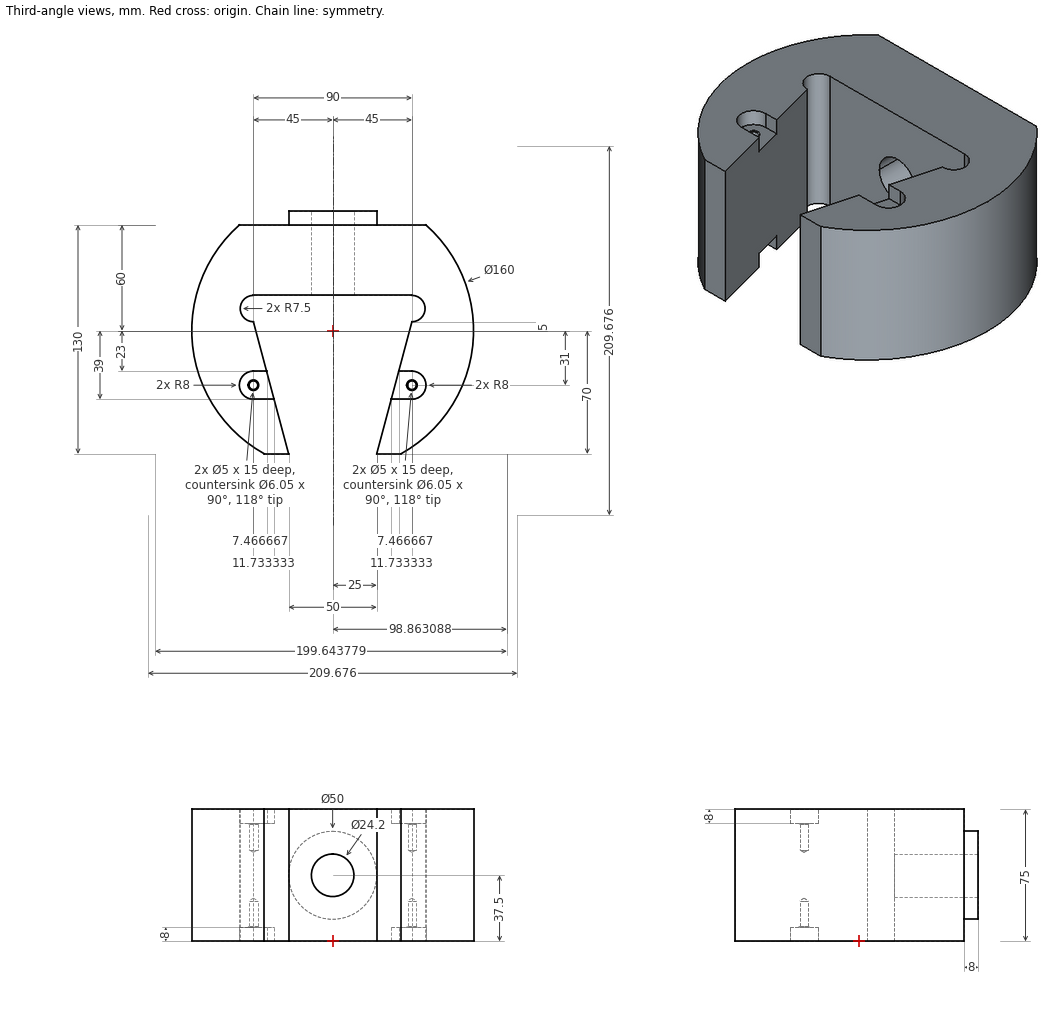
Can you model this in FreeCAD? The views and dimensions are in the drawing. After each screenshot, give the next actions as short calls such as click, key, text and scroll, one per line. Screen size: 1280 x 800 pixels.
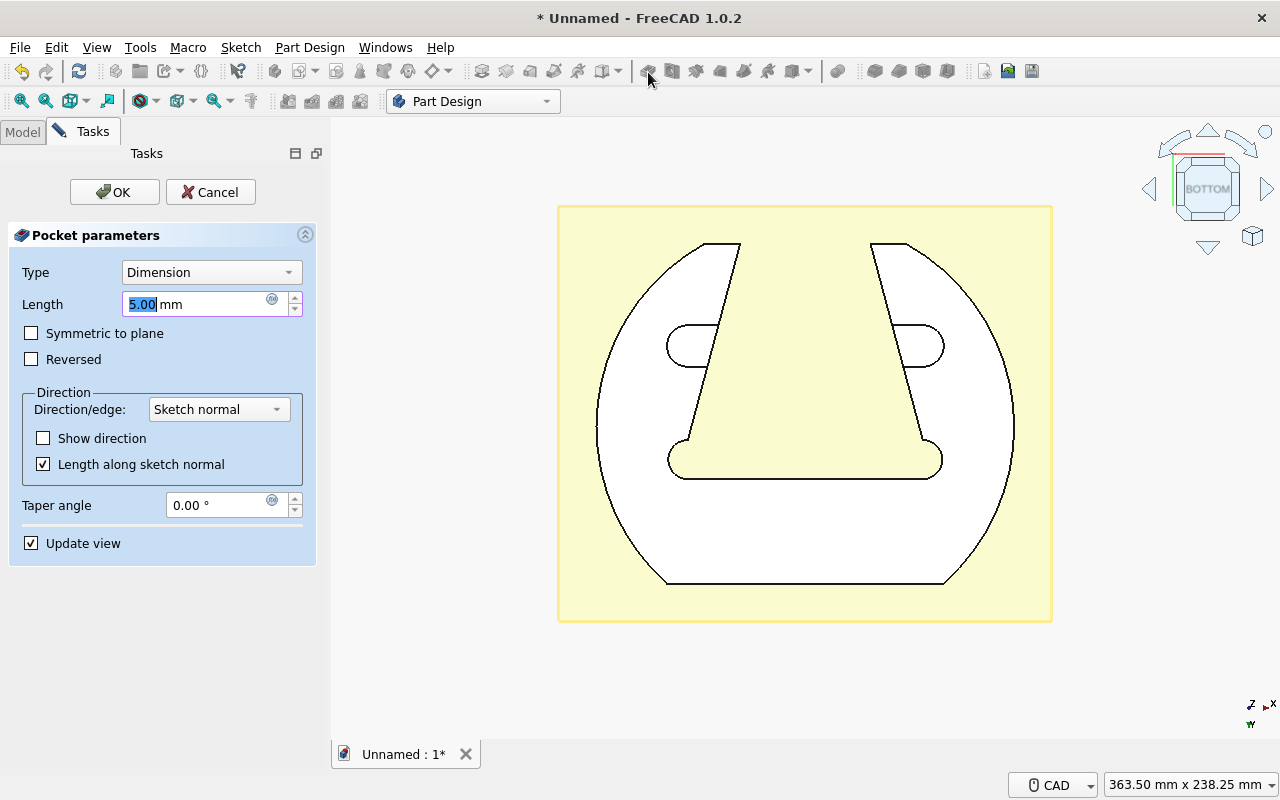
text(8)
key(Tab)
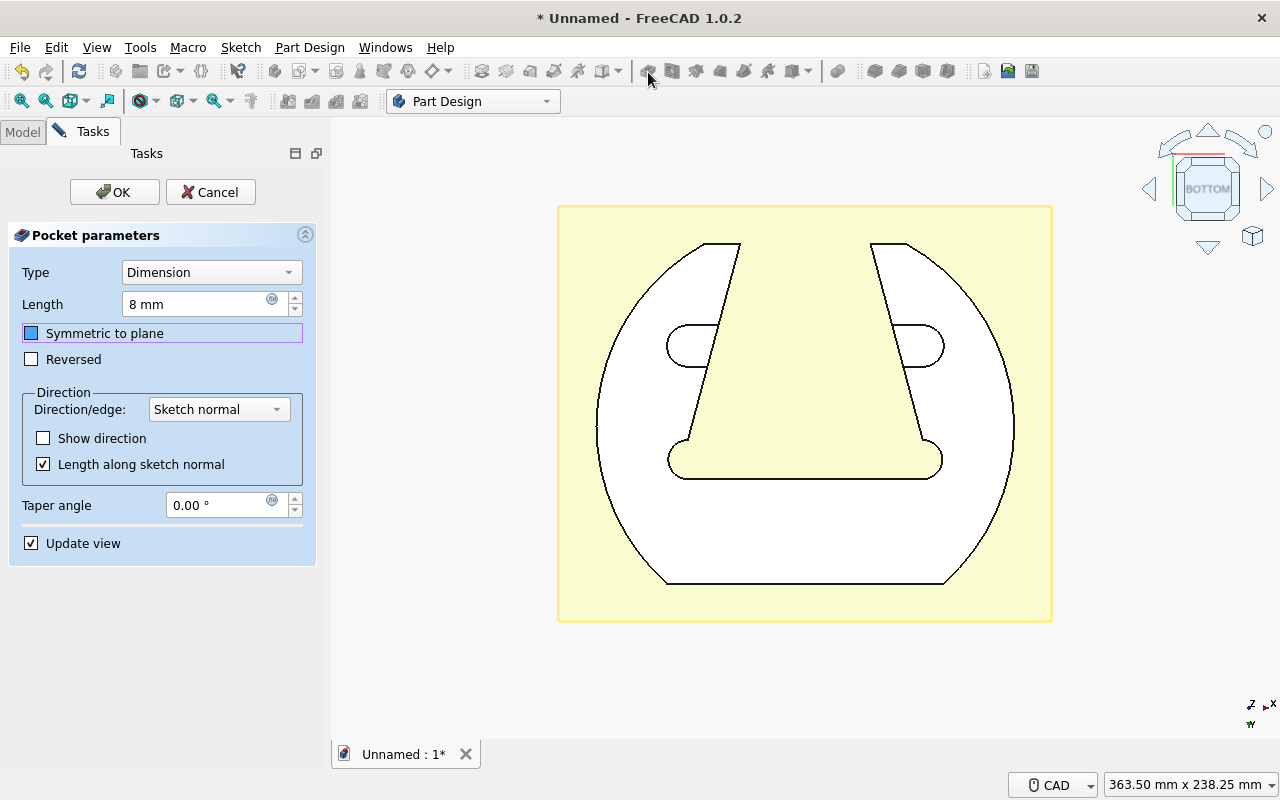
click(30, 359)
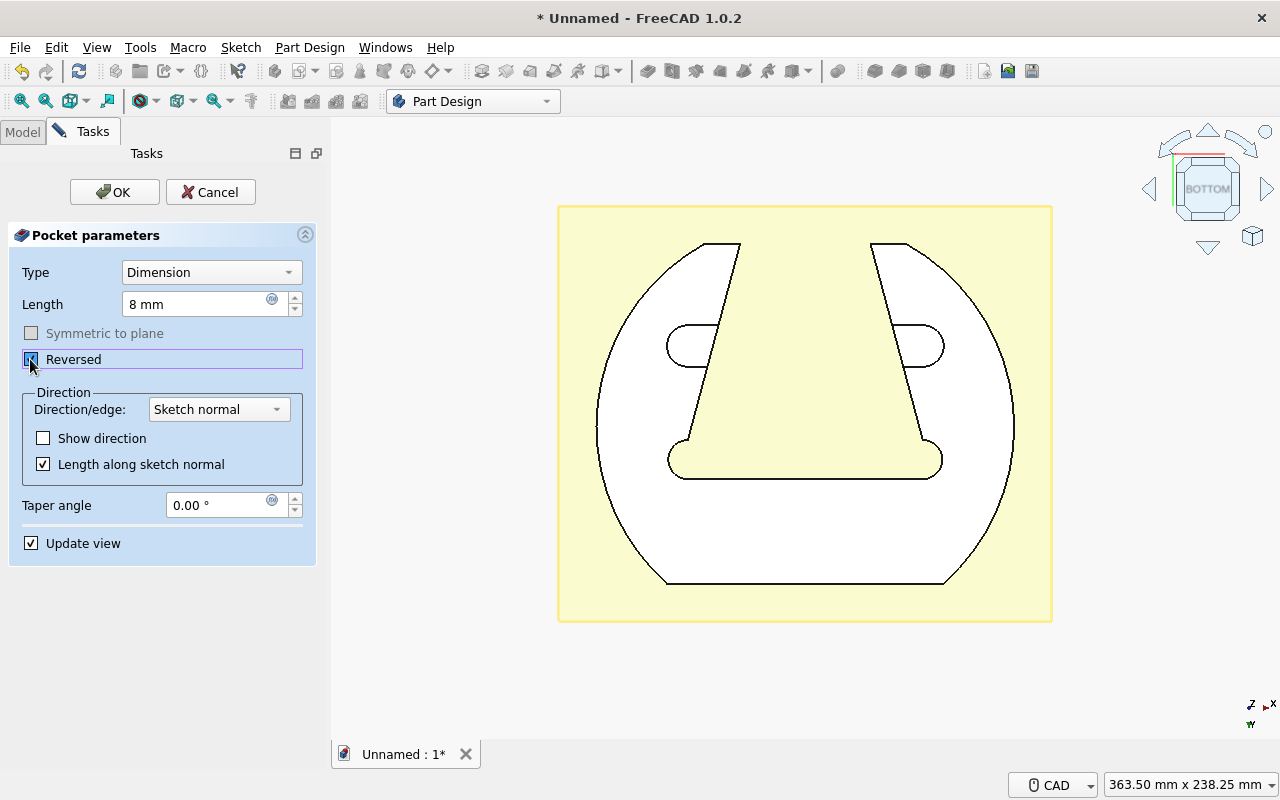
click(115, 192)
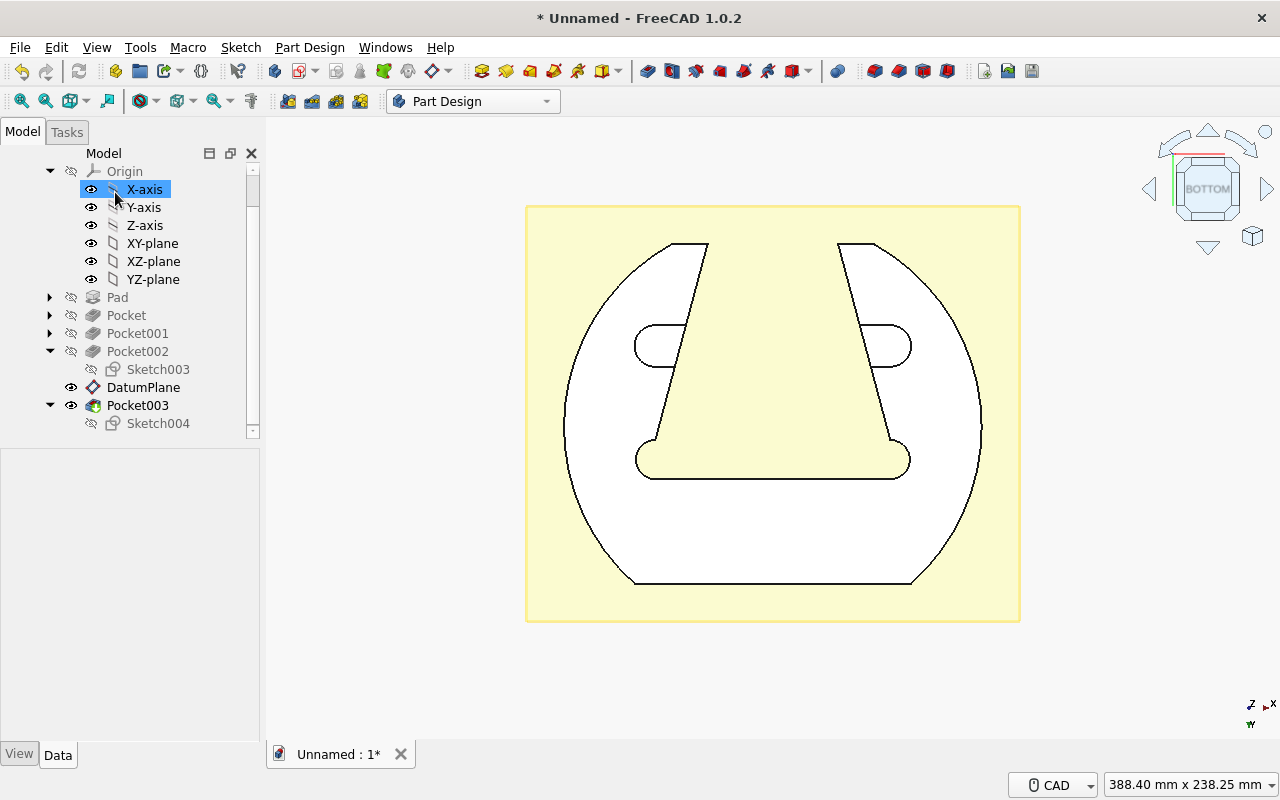
click(116, 387)
key(space)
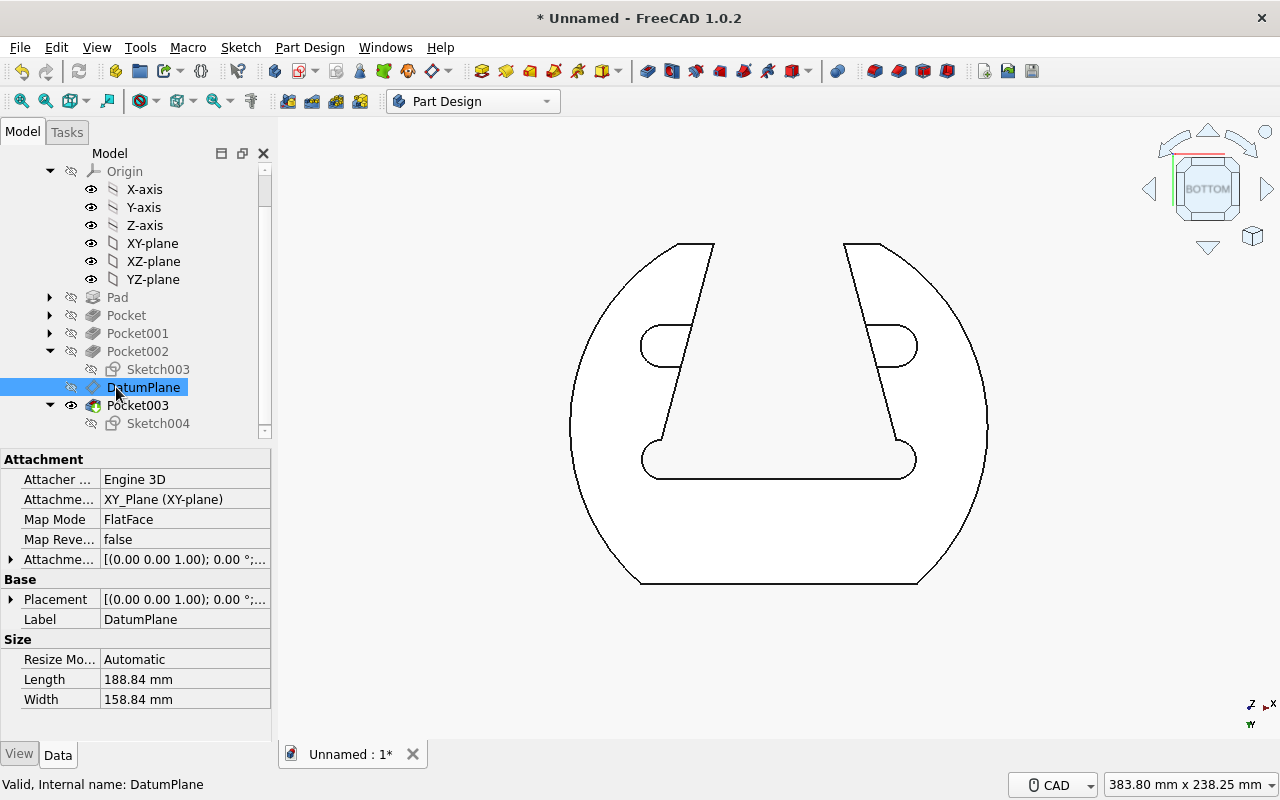
click(666, 345)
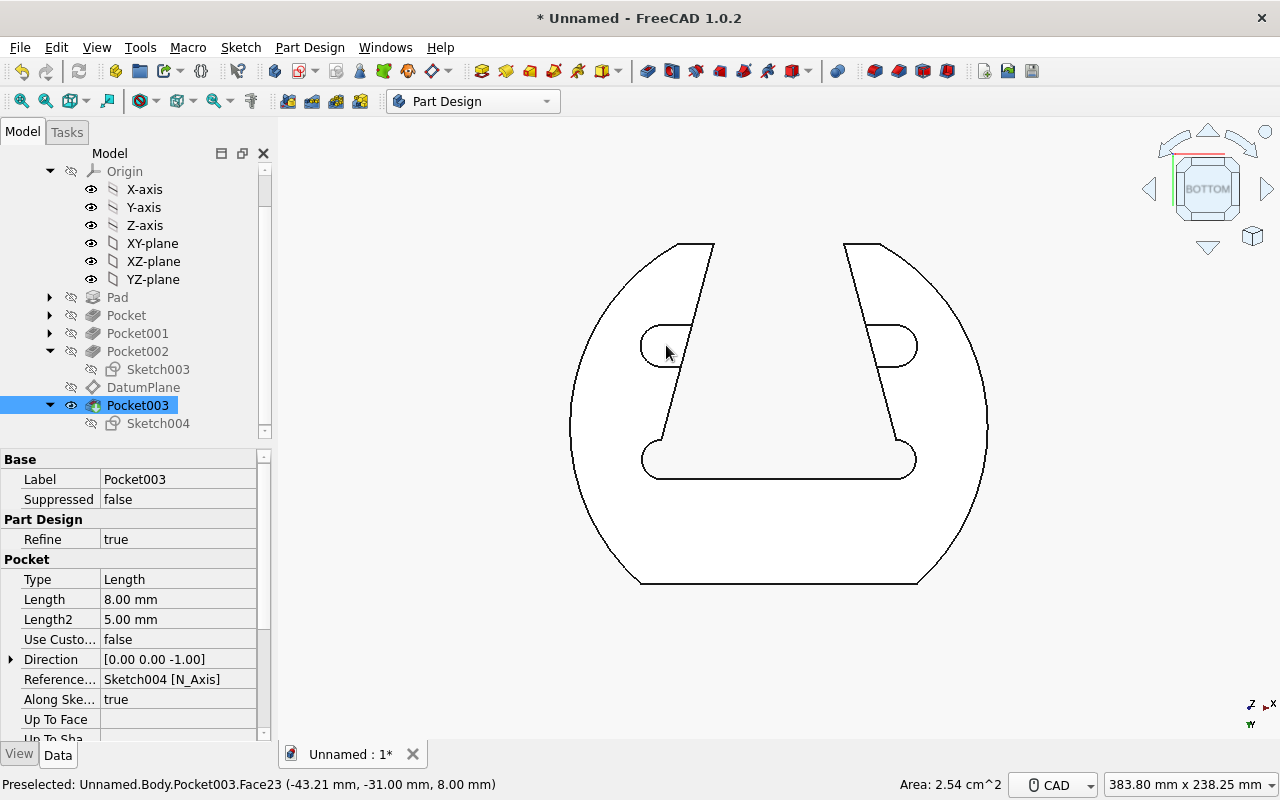
click(300, 72)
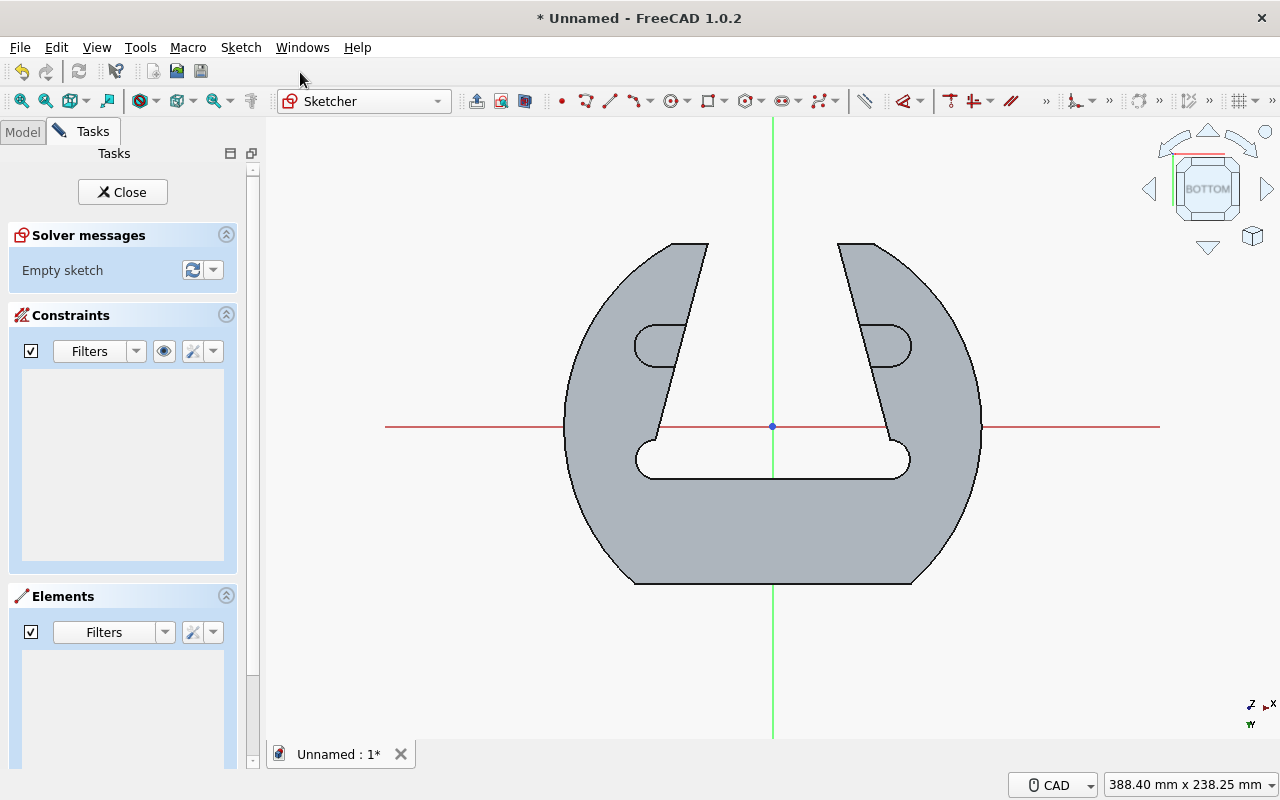
key(q)
key(s)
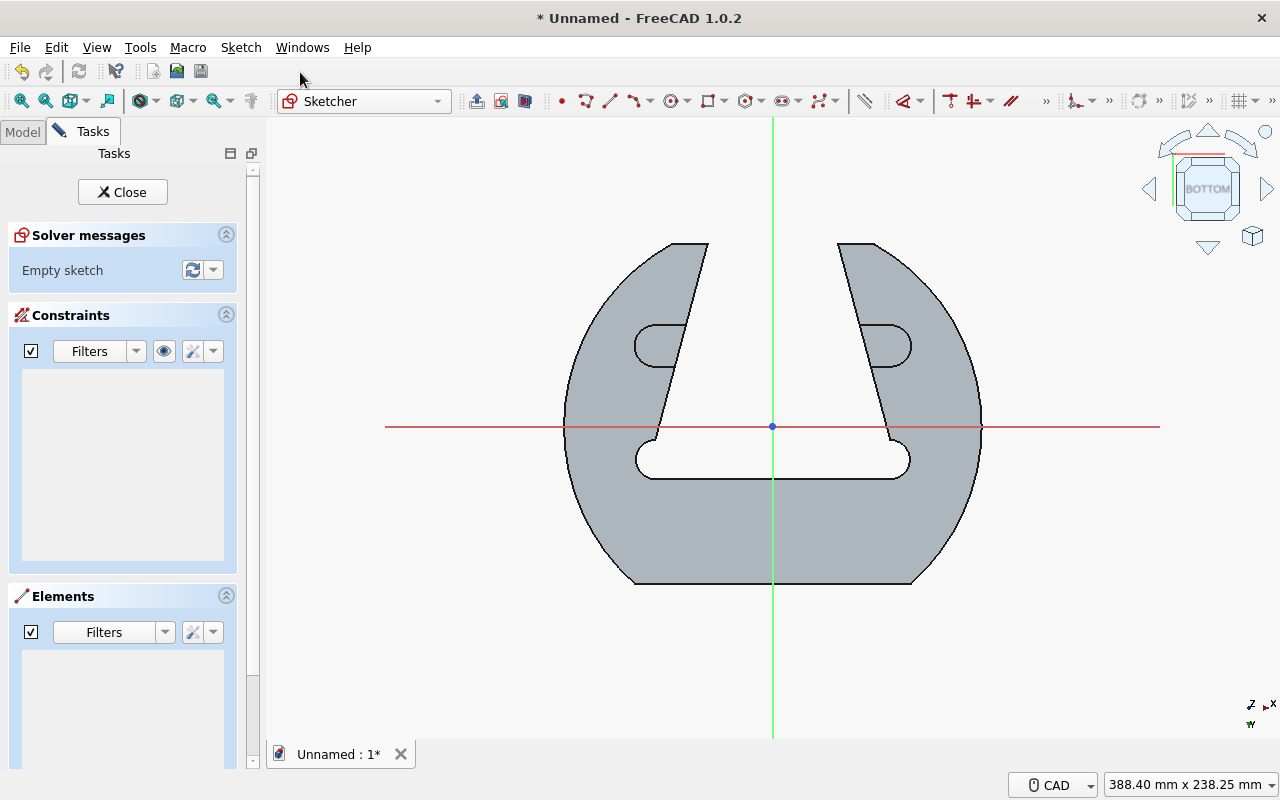
scroll(829, 347, up, 4)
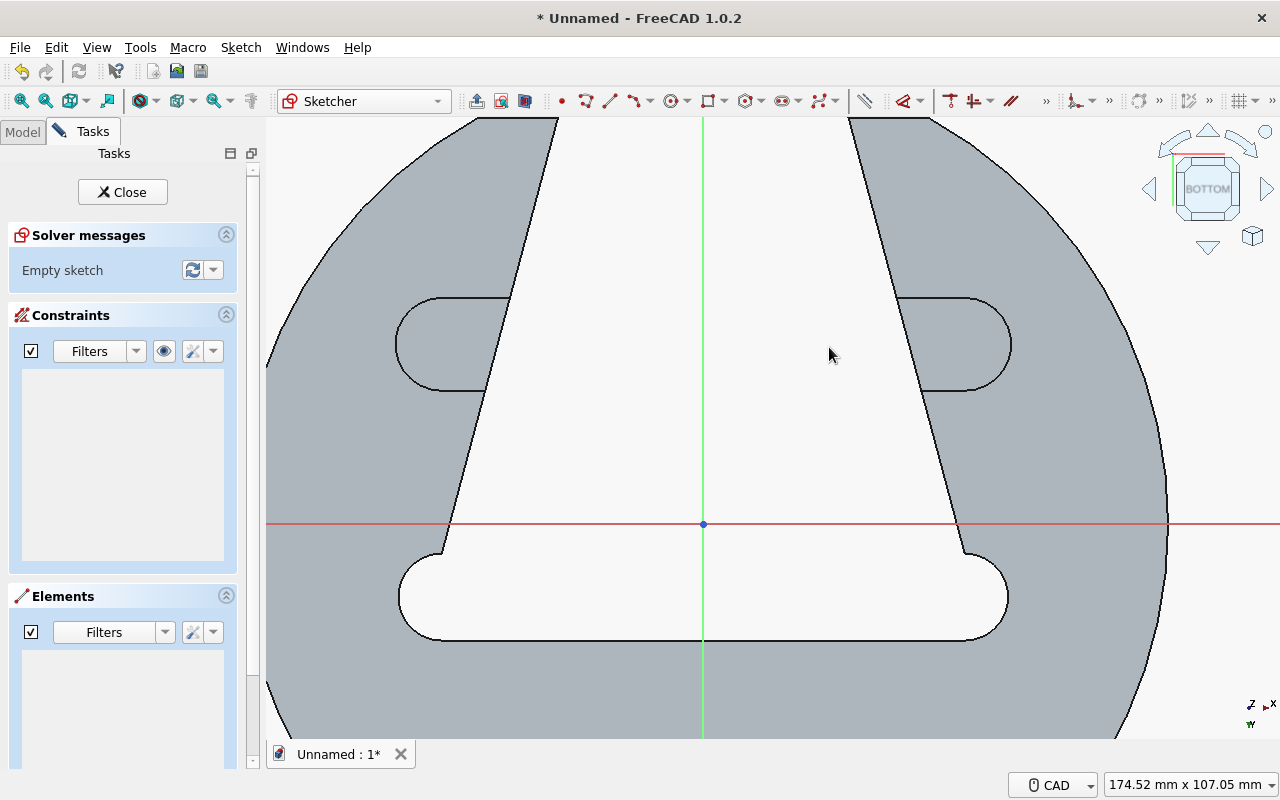
key(g)
key(c)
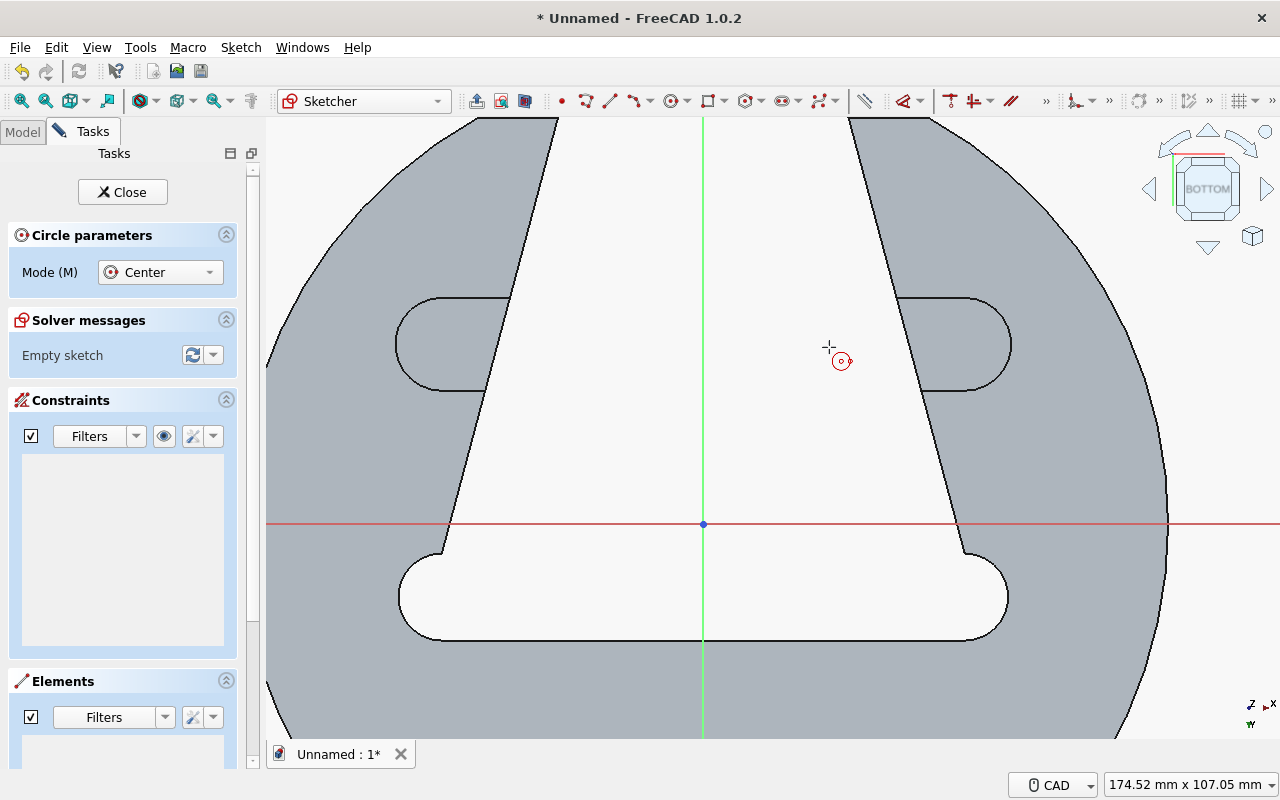
scroll(965, 344, up, 3)